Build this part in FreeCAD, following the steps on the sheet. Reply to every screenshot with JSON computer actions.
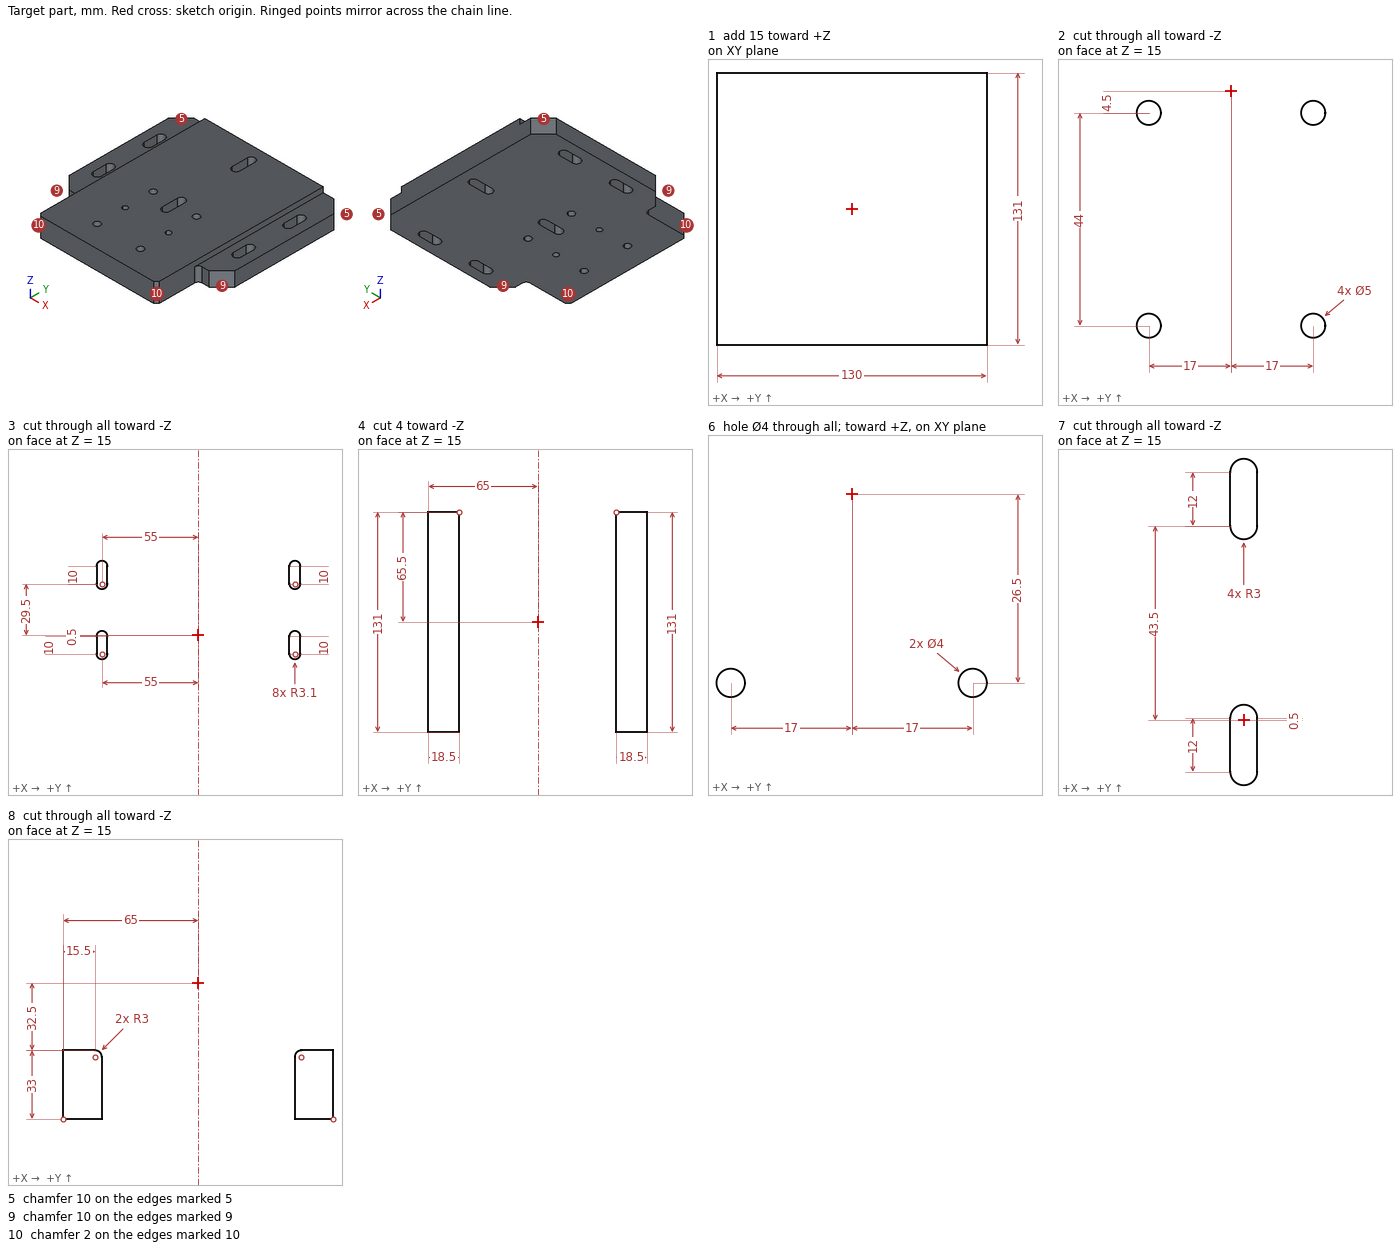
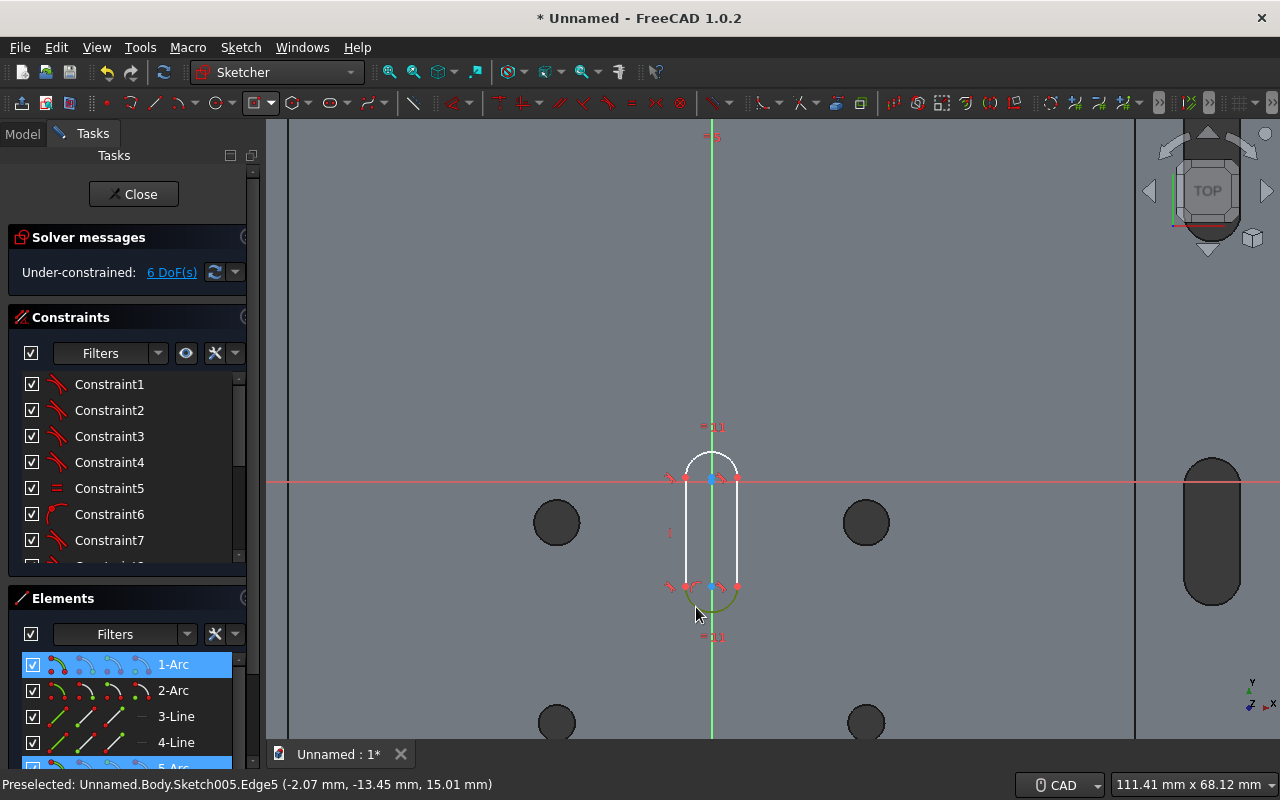
{"action": "key", "text": "e"}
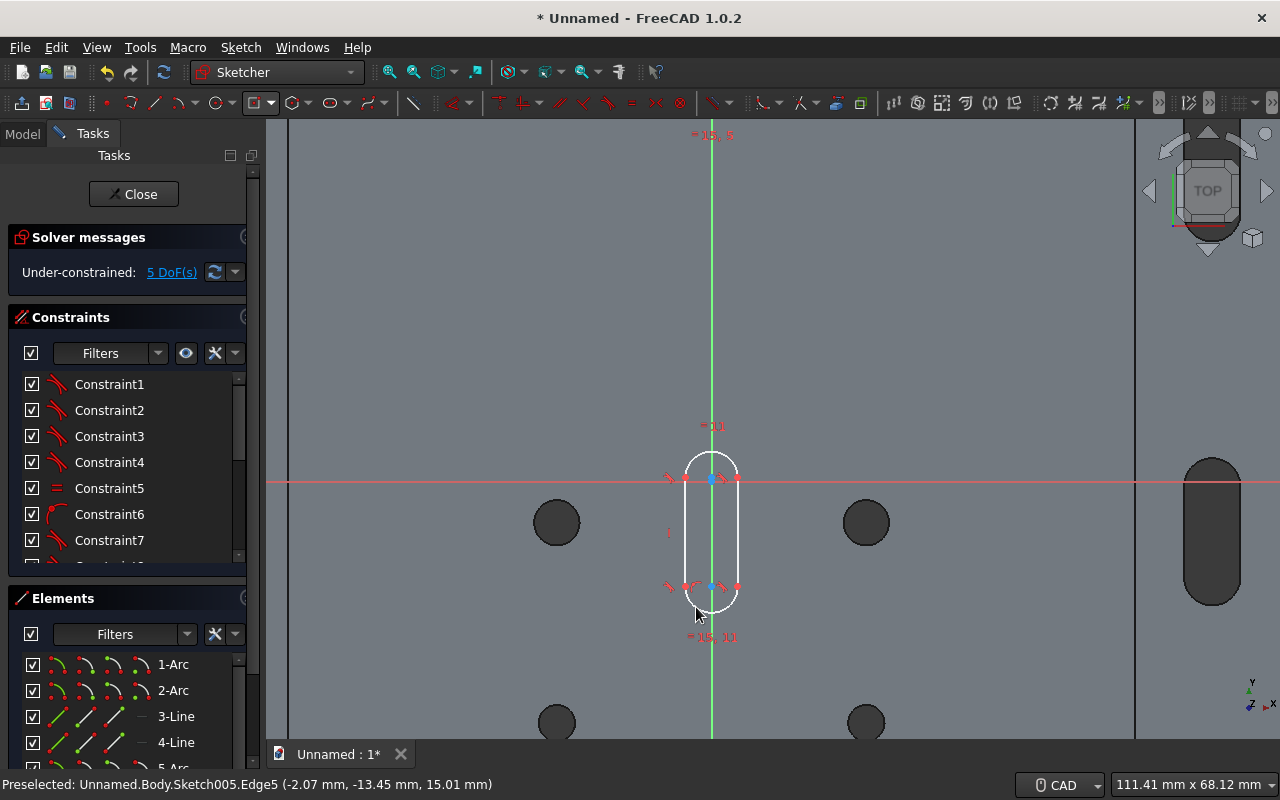
{"action": "left_click", "coordinate": [452, 104]}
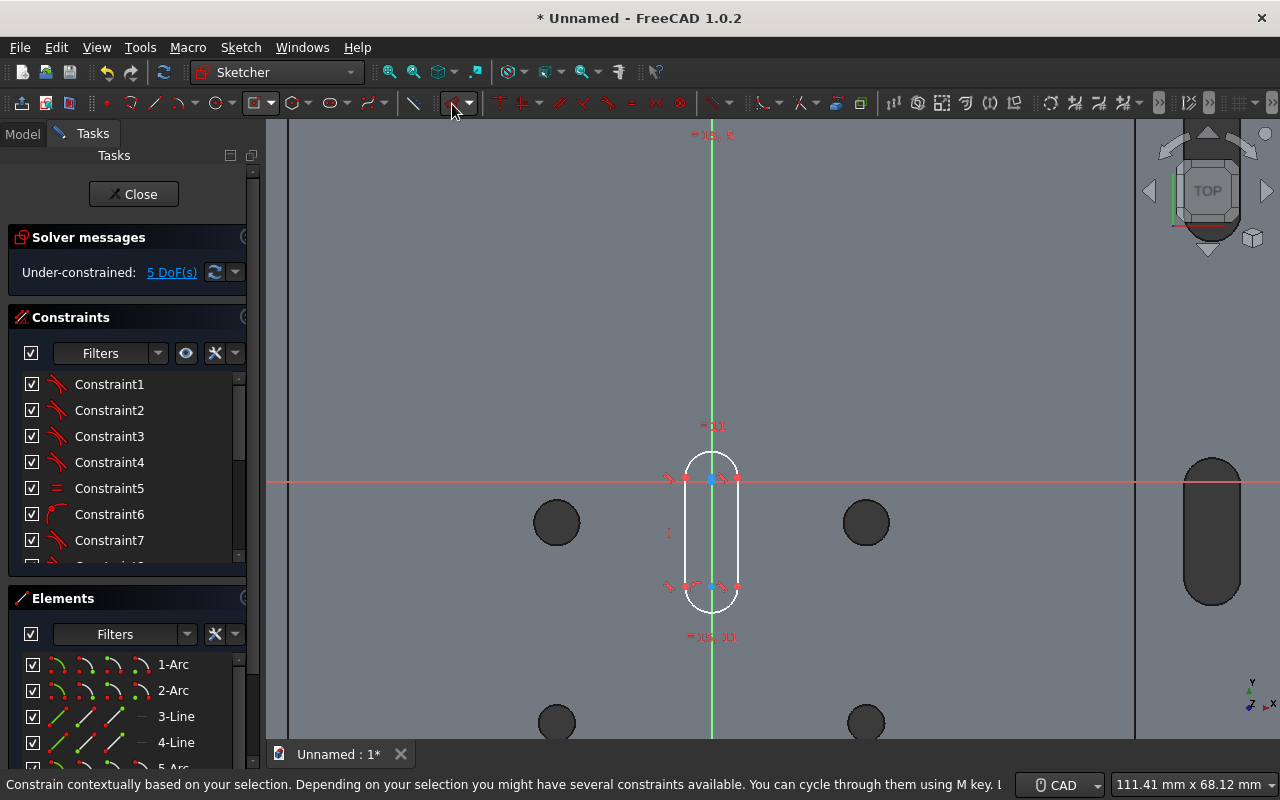
{"action": "scroll", "coordinate": [696, 608], "scroll_direction": "down", "scroll_amount": 3}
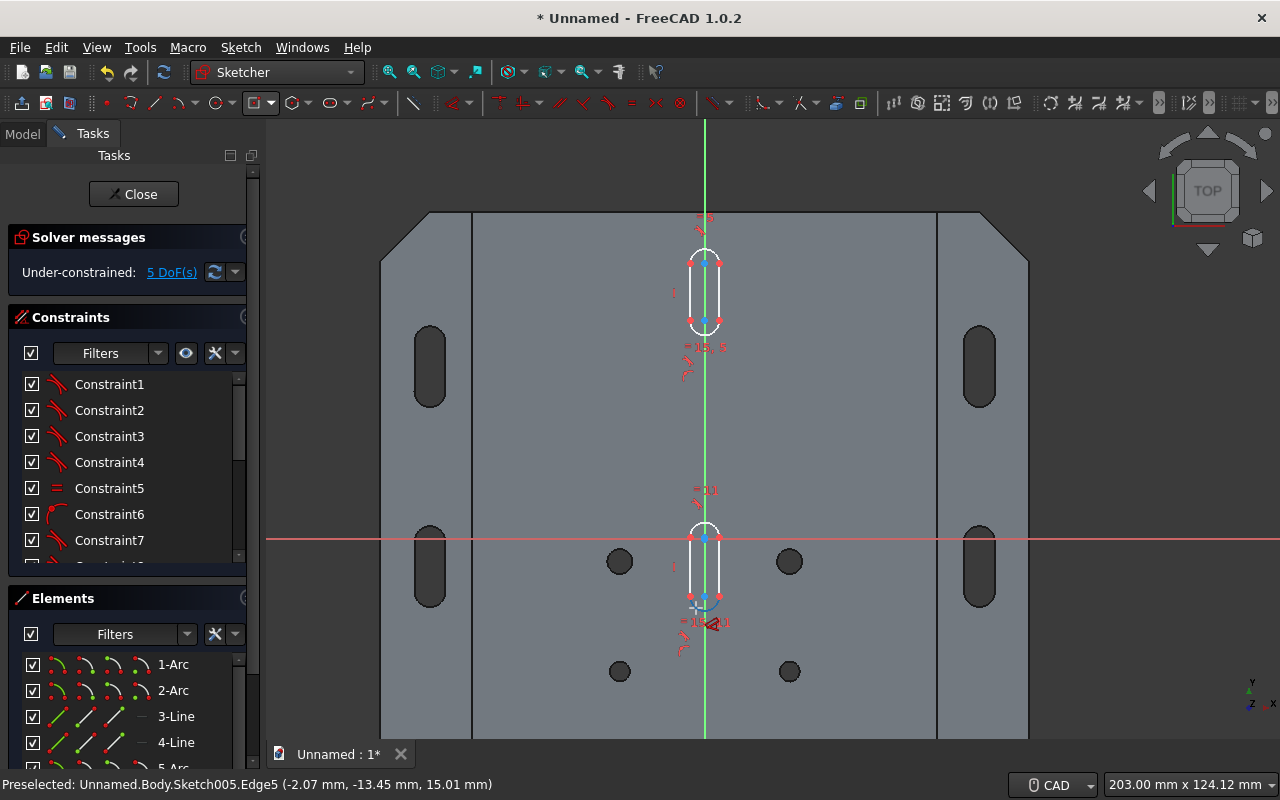
{"action": "scroll", "coordinate": [696, 333], "scroll_direction": "up", "scroll_amount": 5}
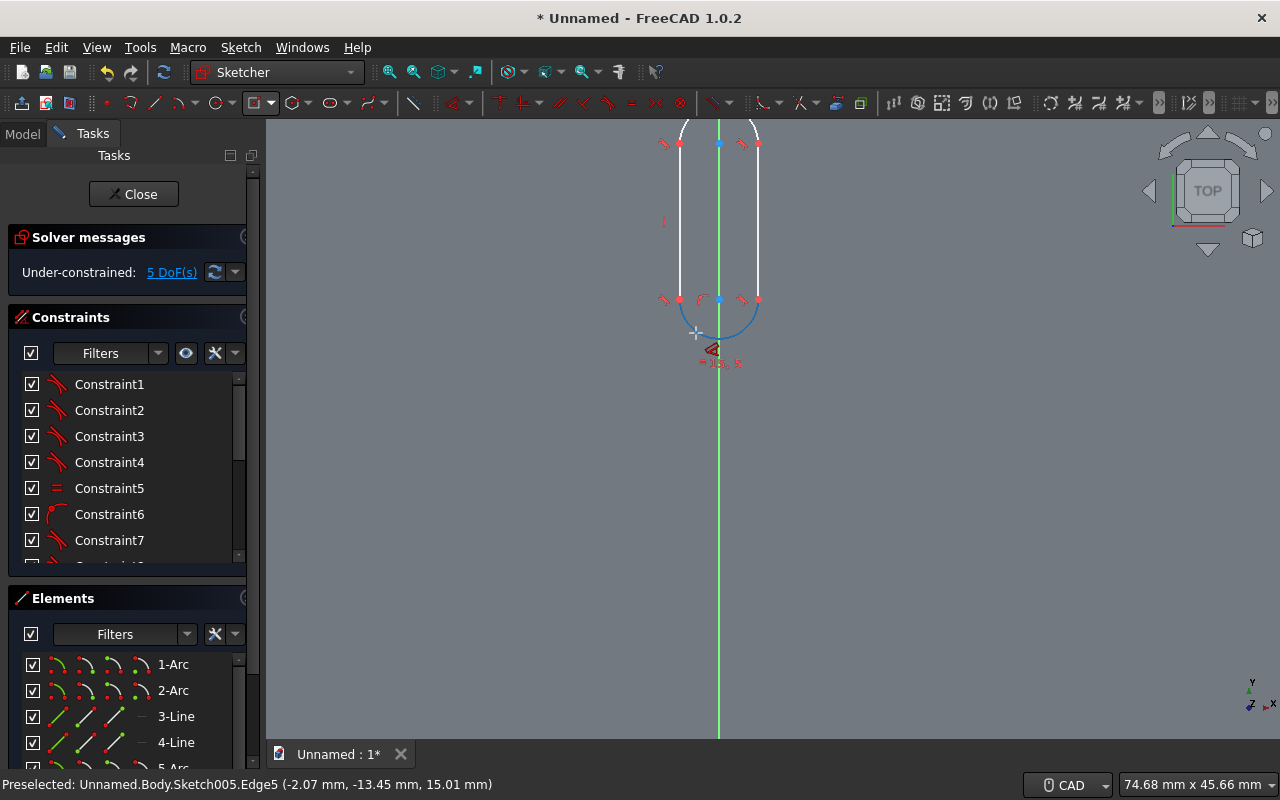
{"action": "left_click", "coordinate": [696, 331]}
{"action": "left_click", "coordinate": [677, 357]}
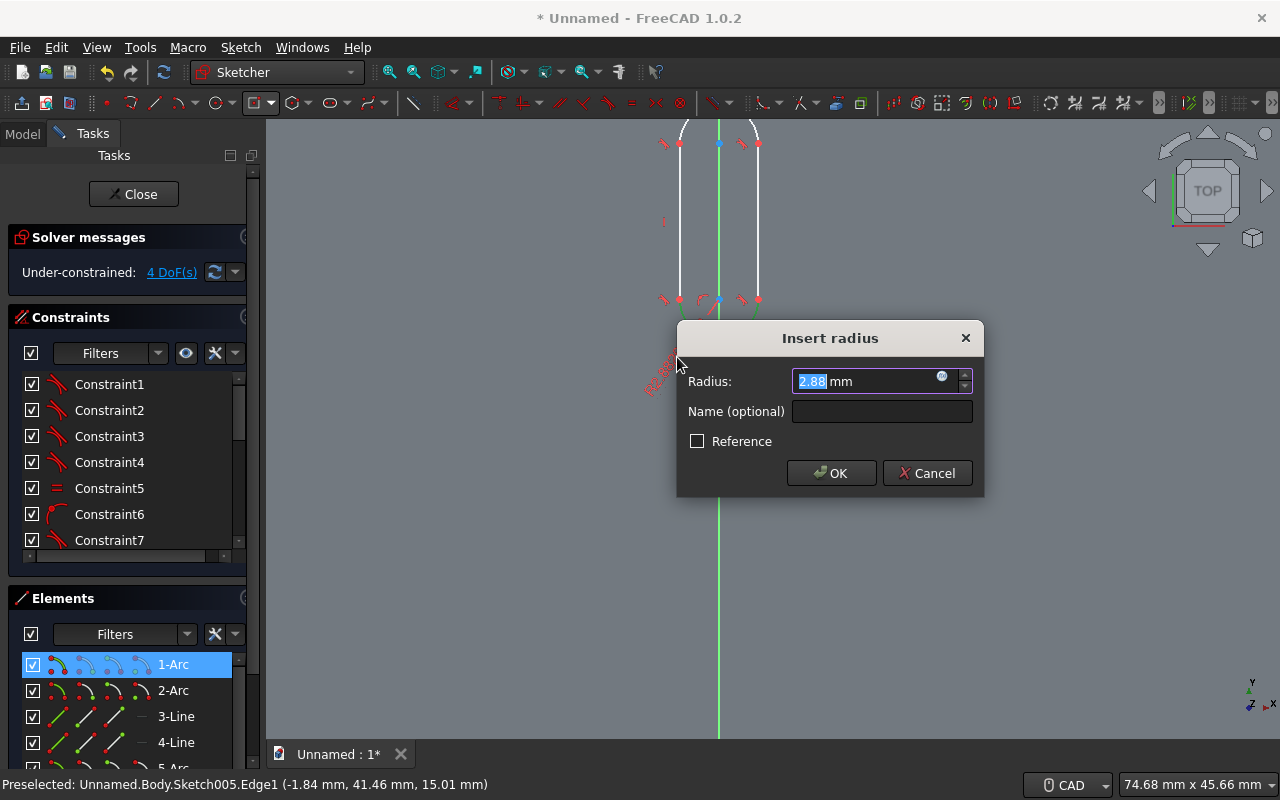
{"action": "type", "text": "3"}
{"action": "key", "text": "Return"}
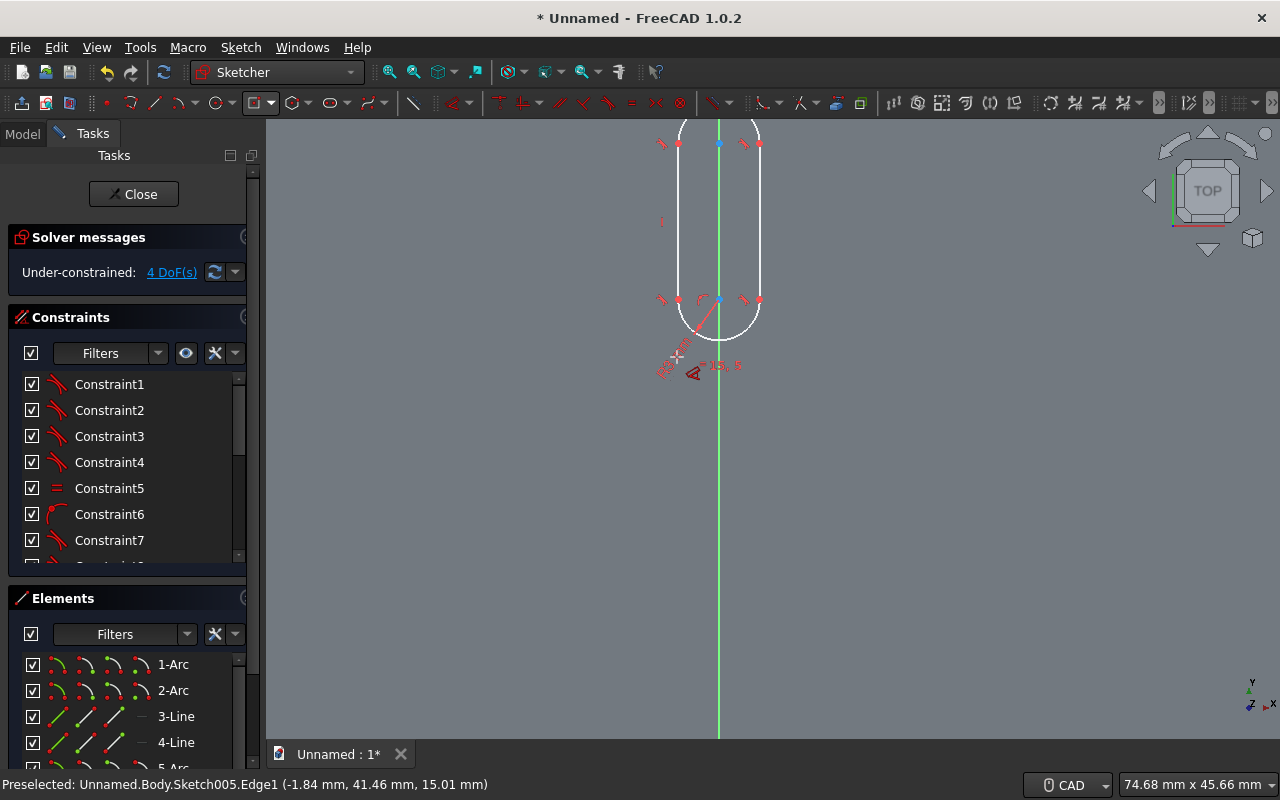
{"action": "left_click", "coordinate": [678, 253]}
{"action": "left_click", "coordinate": [644, 223]}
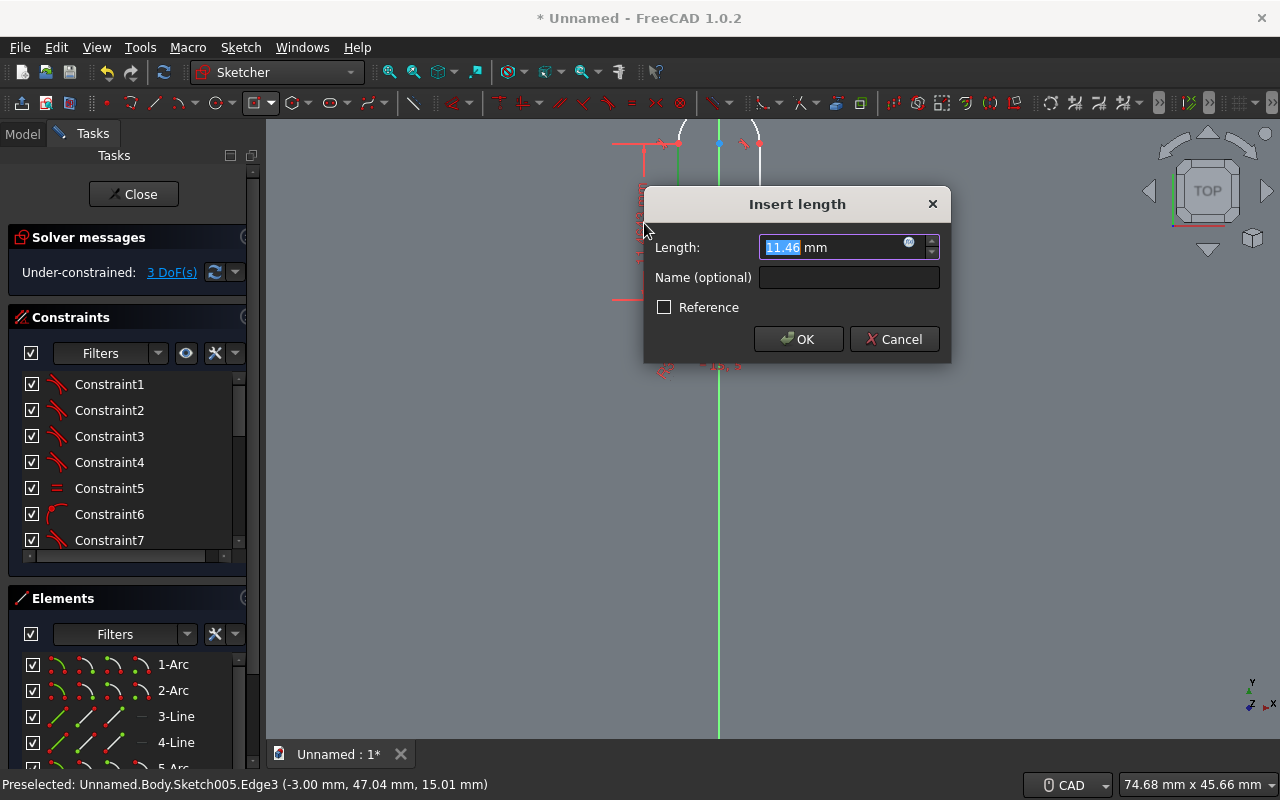
{"action": "type", "text": "12"}
{"action": "key", "text": "Return"}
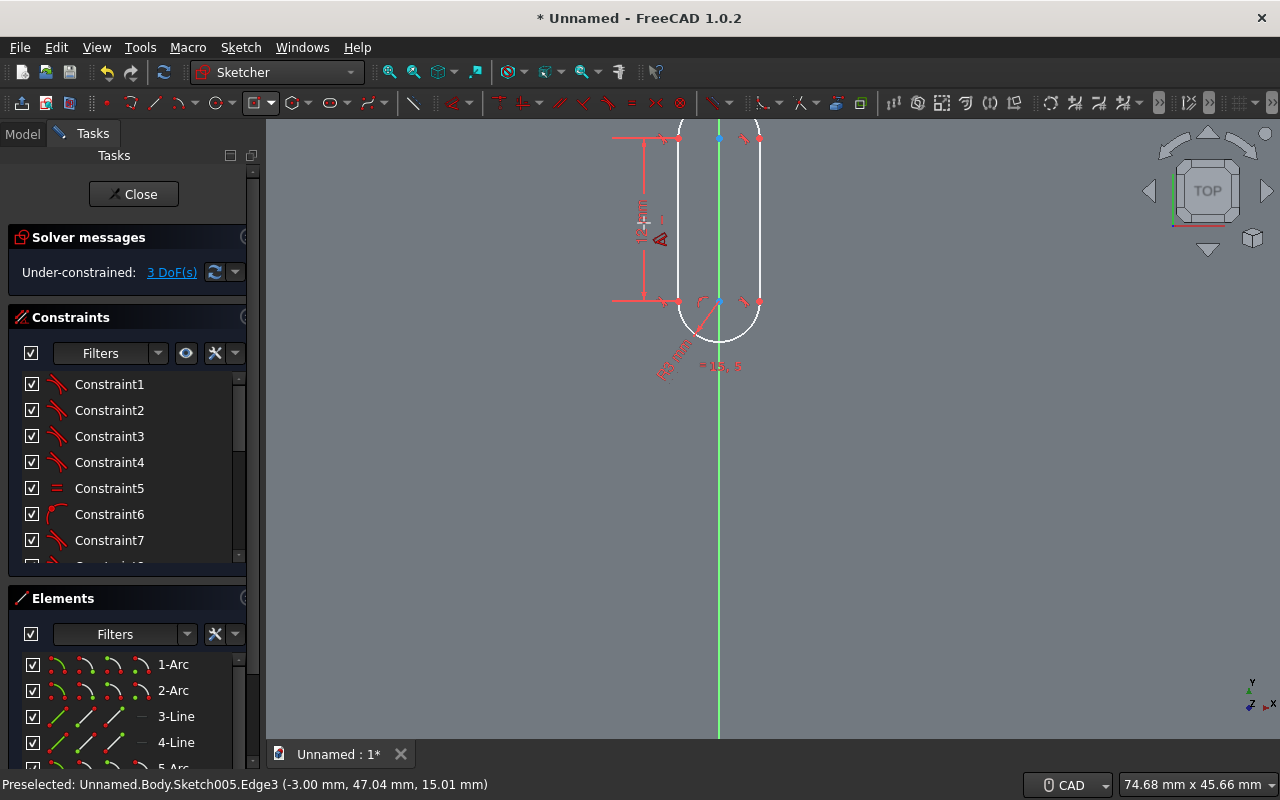
{"action": "scroll", "coordinate": [696, 333], "scroll_direction": "down", "scroll_amount": 5}